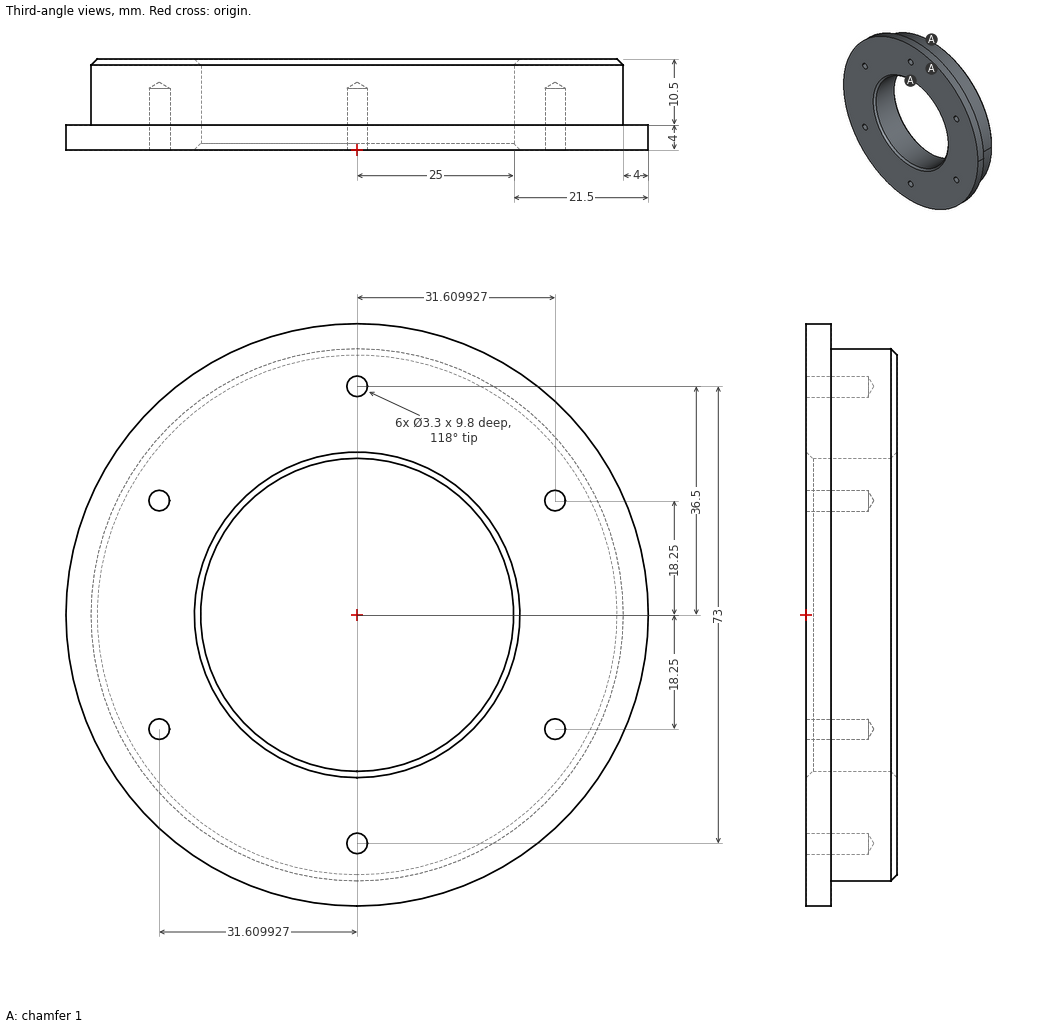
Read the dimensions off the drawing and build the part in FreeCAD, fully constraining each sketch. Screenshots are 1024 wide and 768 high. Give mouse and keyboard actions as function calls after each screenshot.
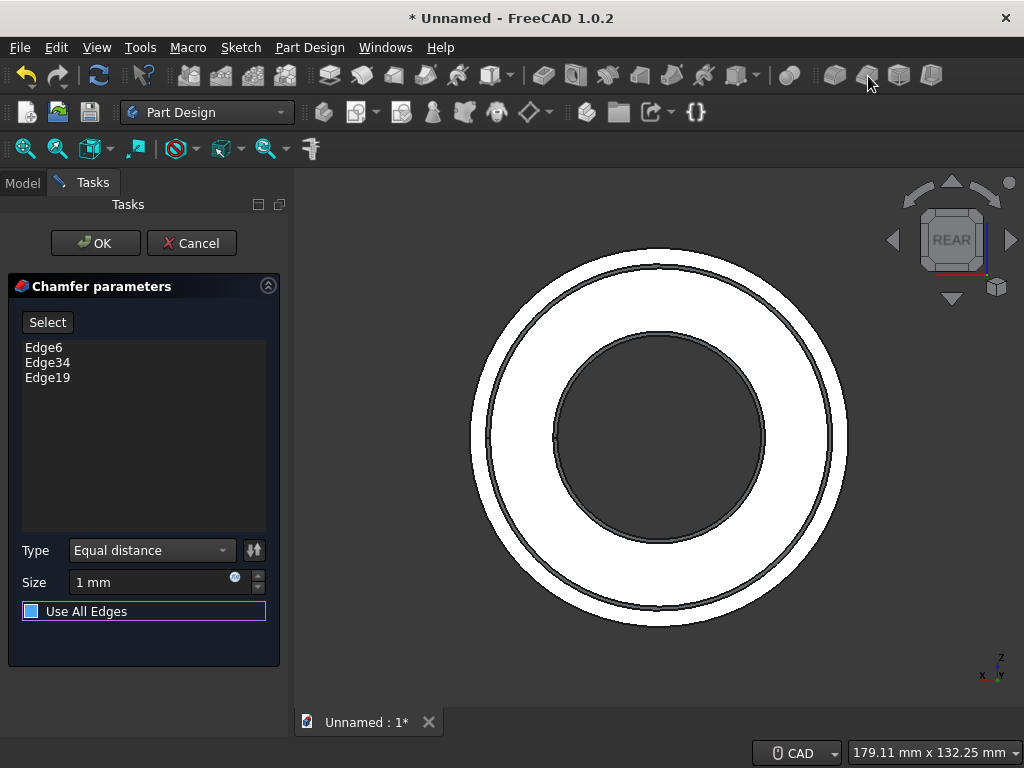
click(96, 243)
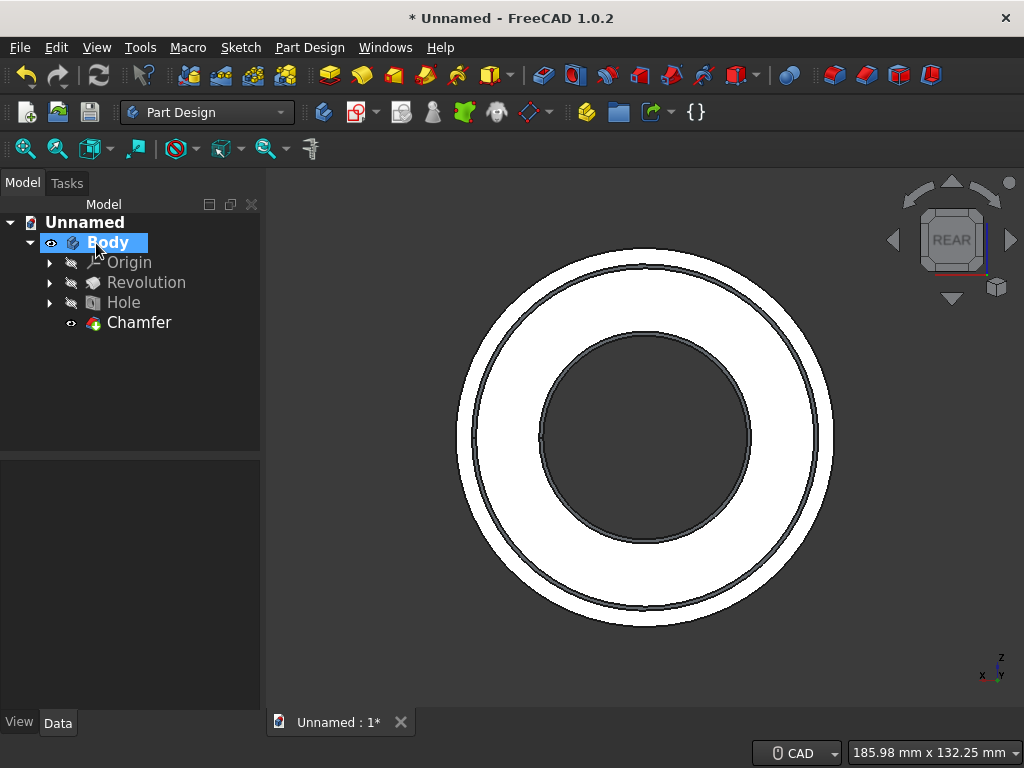
key(0)